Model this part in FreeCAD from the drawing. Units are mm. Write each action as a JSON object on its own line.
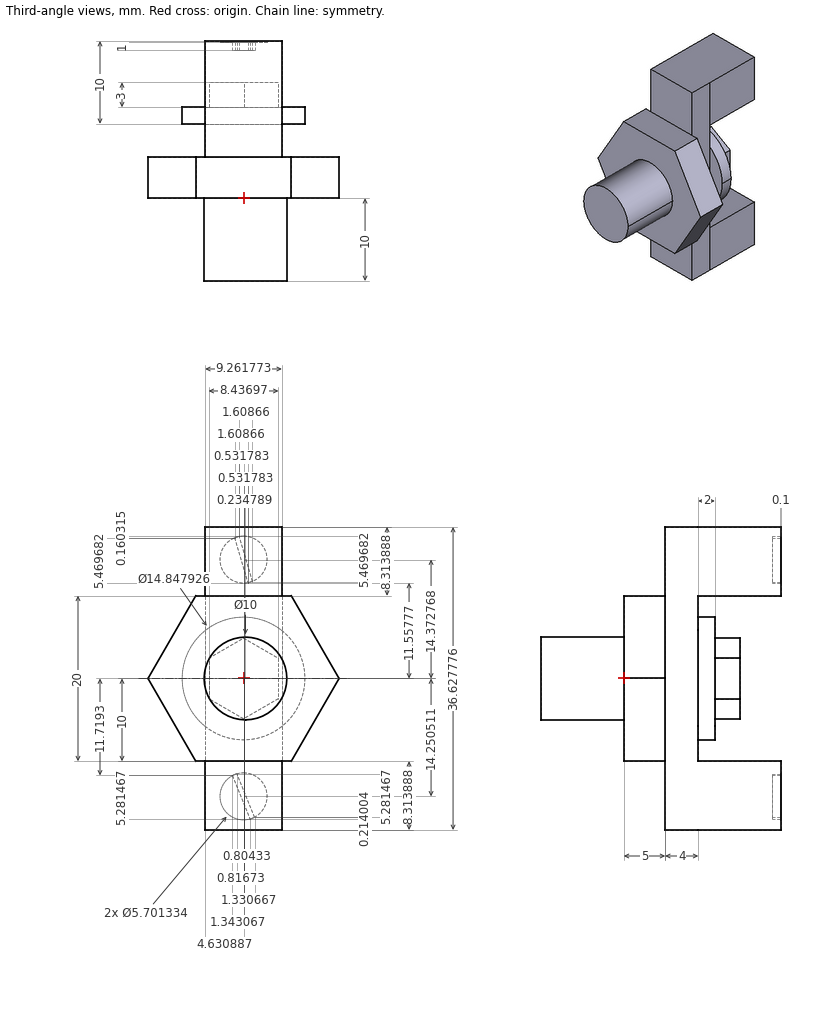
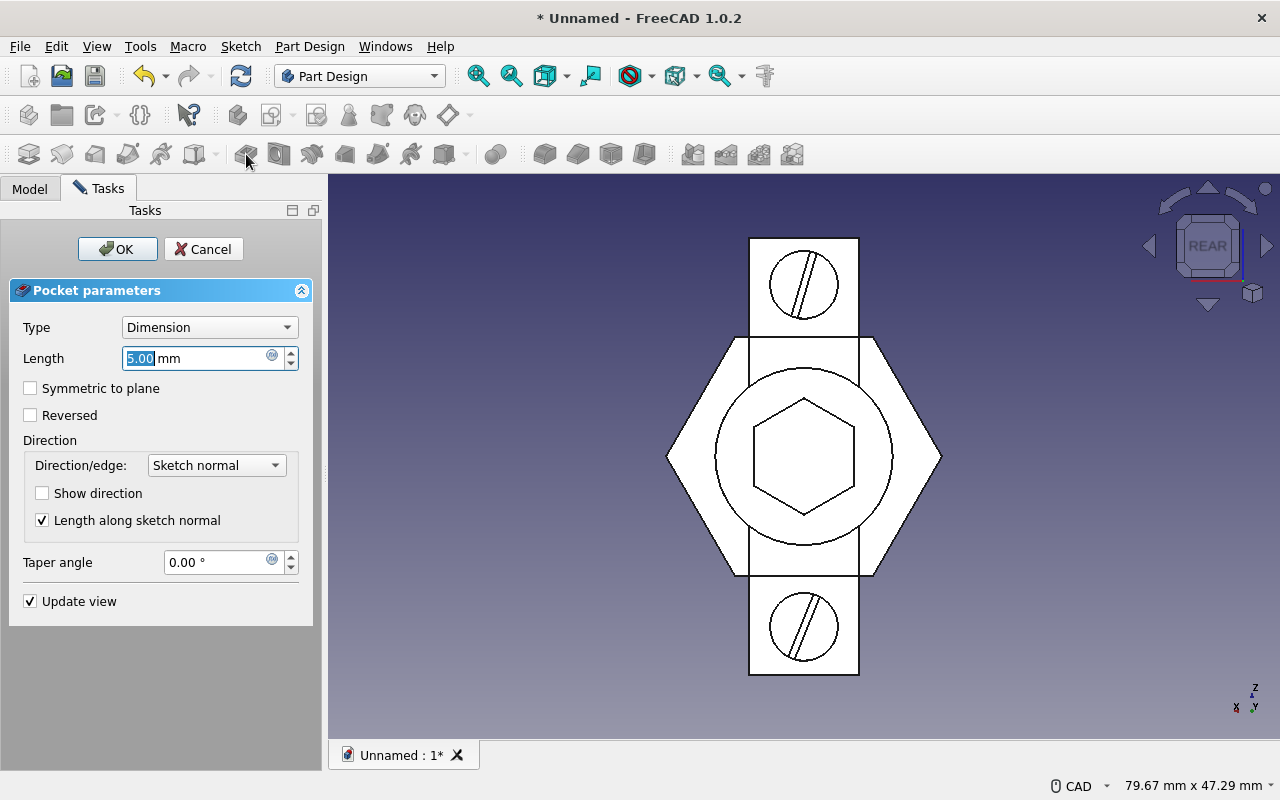
{"action": "type", "text": "1"}
{"action": "key", "text": "Tab"}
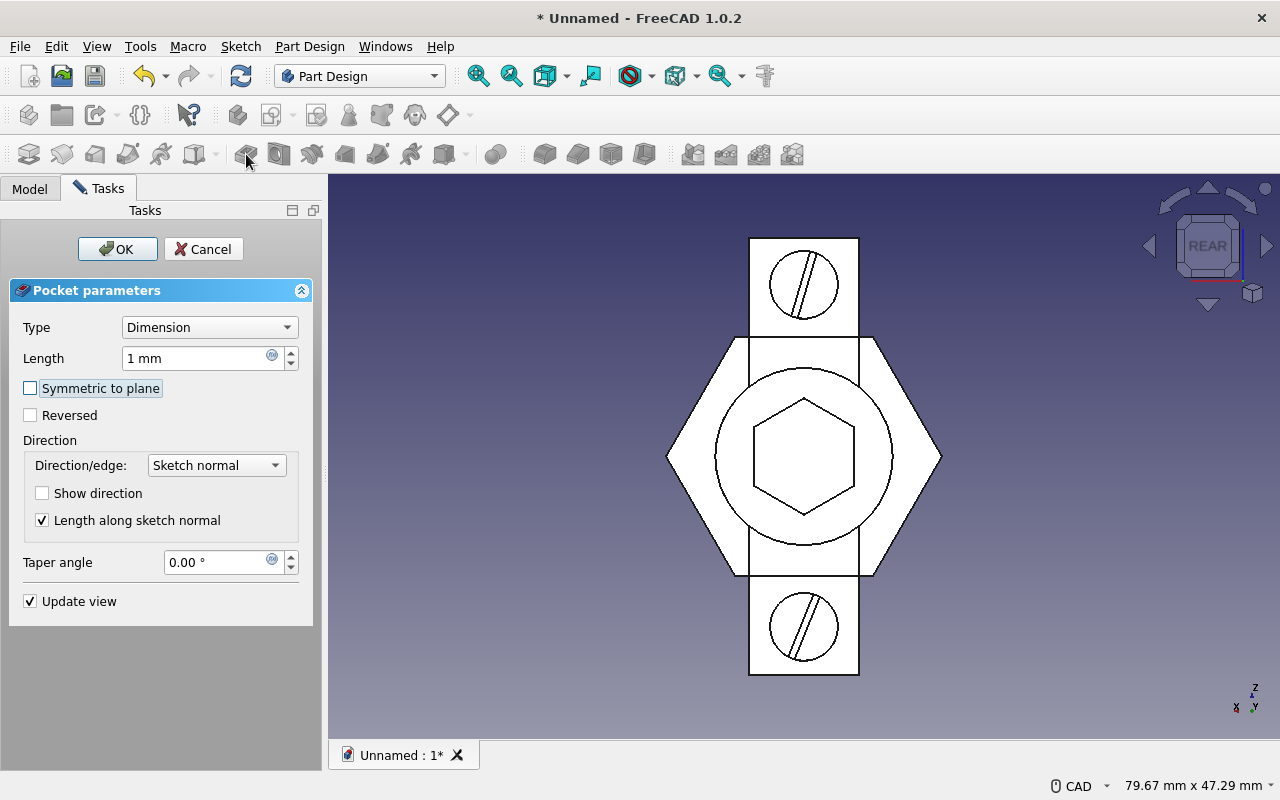
{"action": "left_click", "coordinate": [118, 249]}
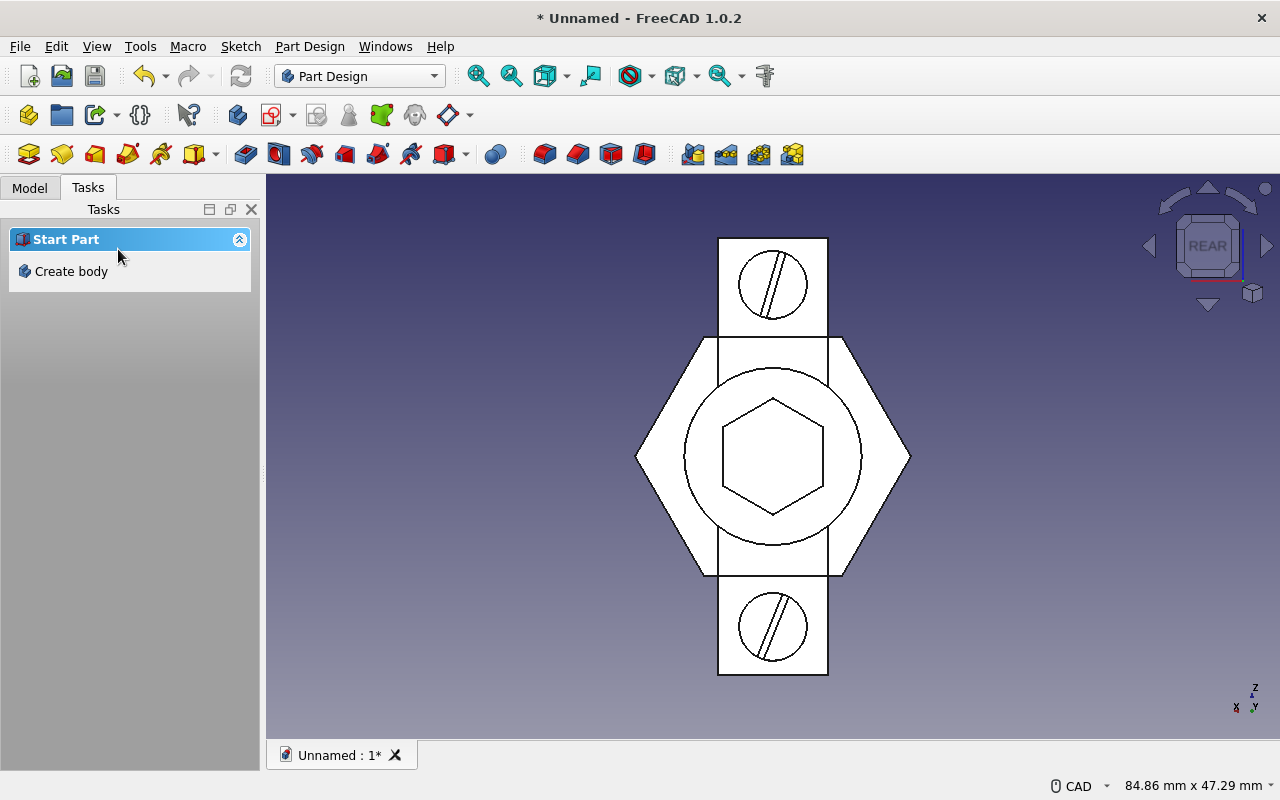
{"action": "key", "text": "0"}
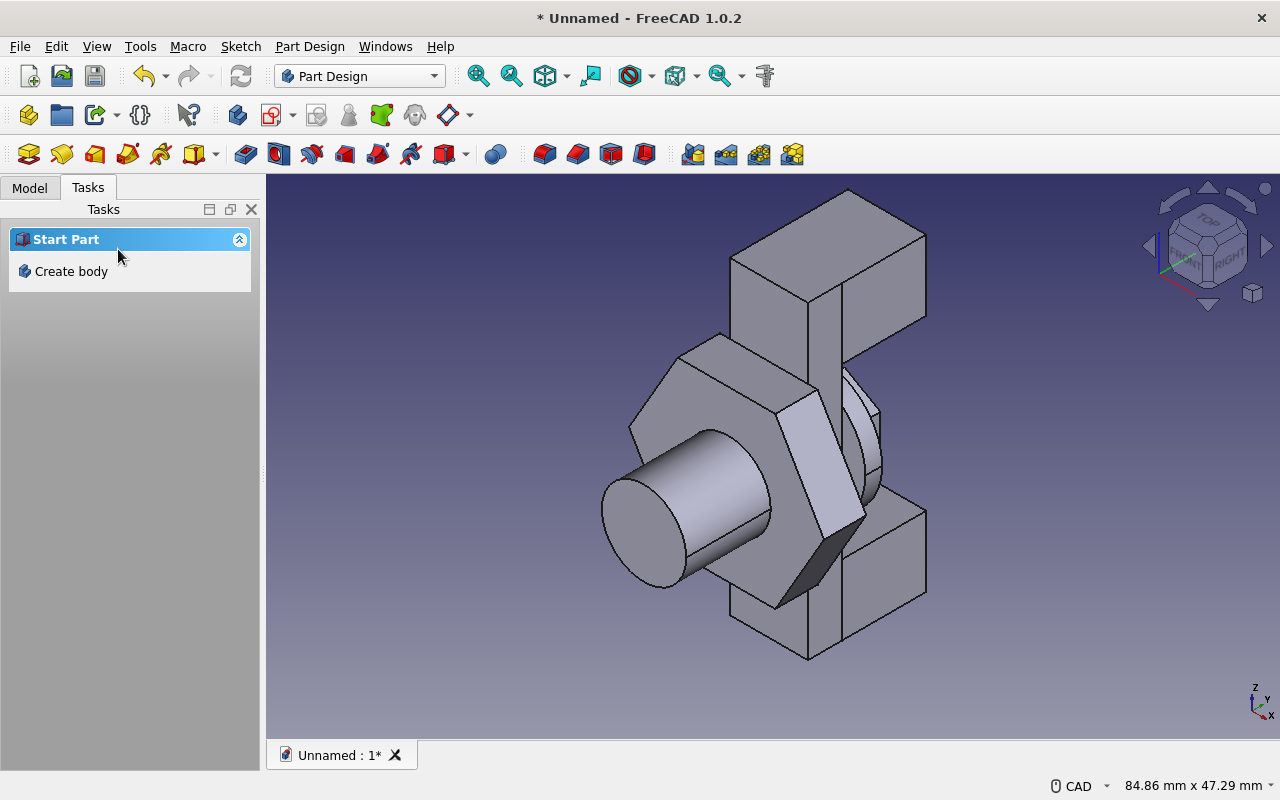
{"action": "left_click", "coordinate": [479, 76]}